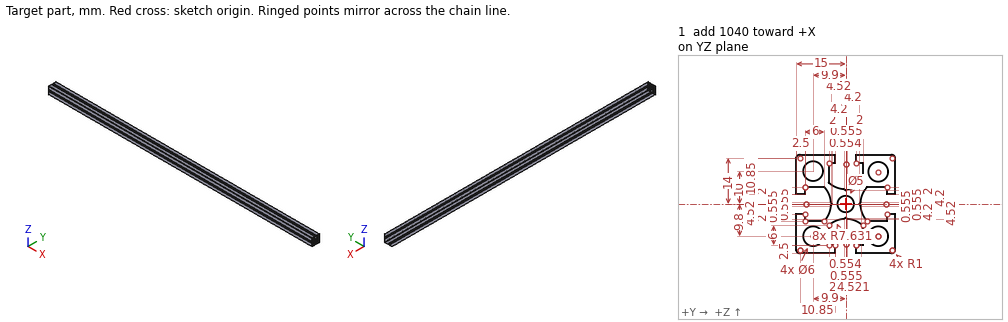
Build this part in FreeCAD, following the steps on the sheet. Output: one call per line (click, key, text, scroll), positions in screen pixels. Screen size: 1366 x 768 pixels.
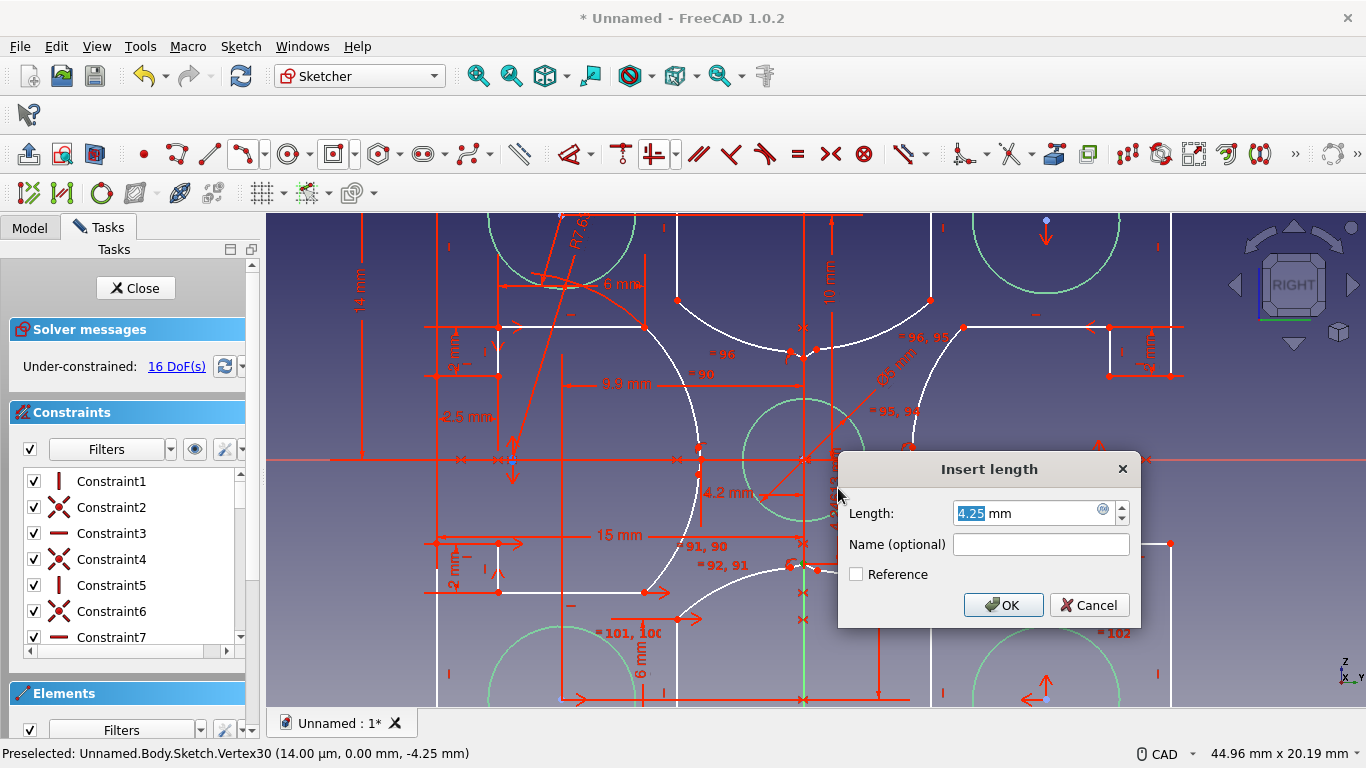
text(4.2)
key(Return)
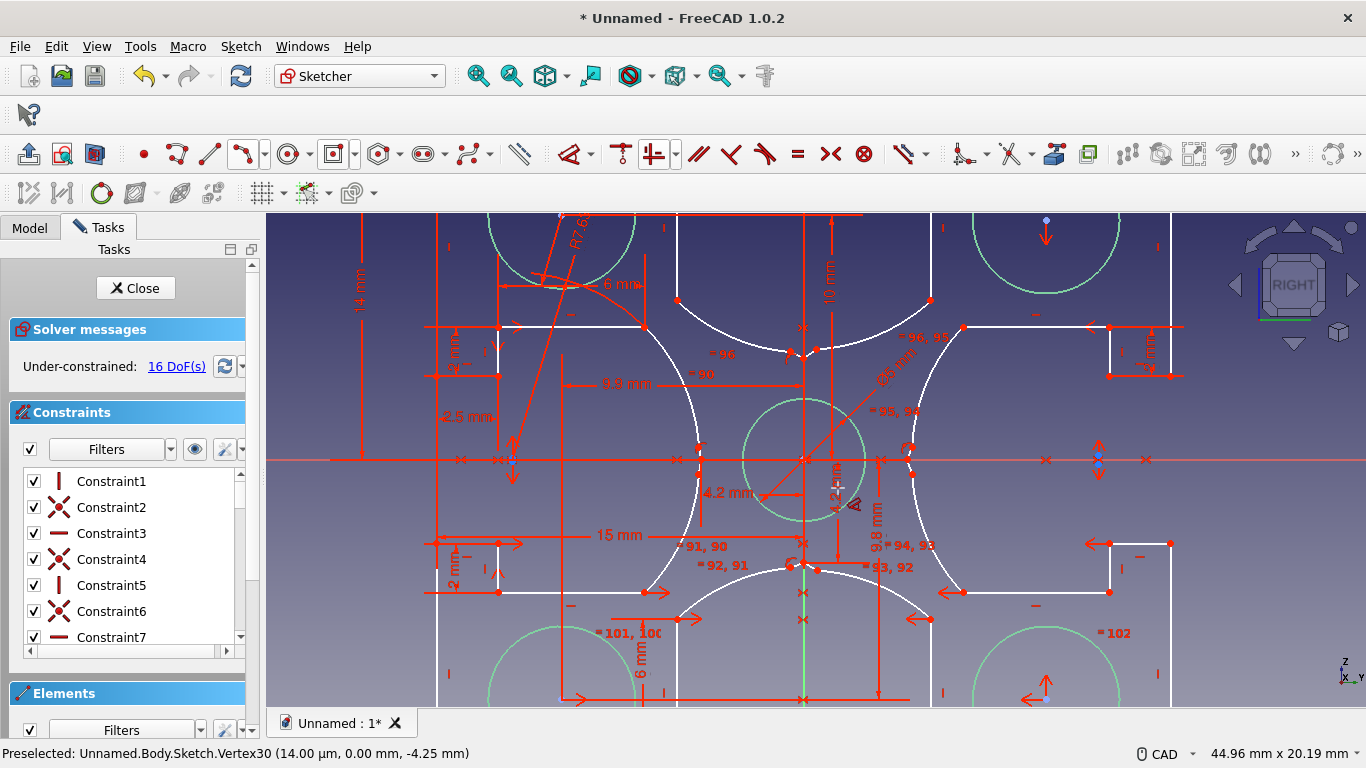
click(907, 460)
click(832, 426)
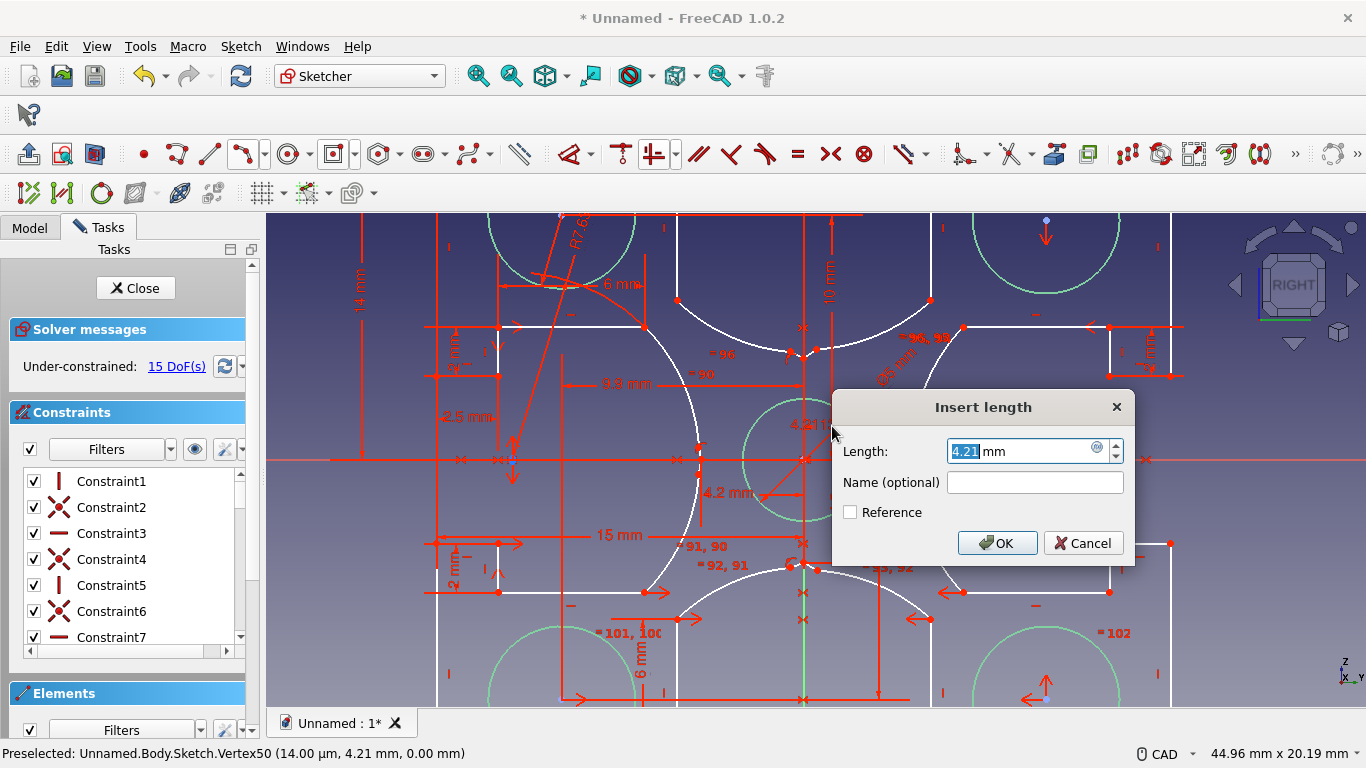
text(4.2)
key(Return)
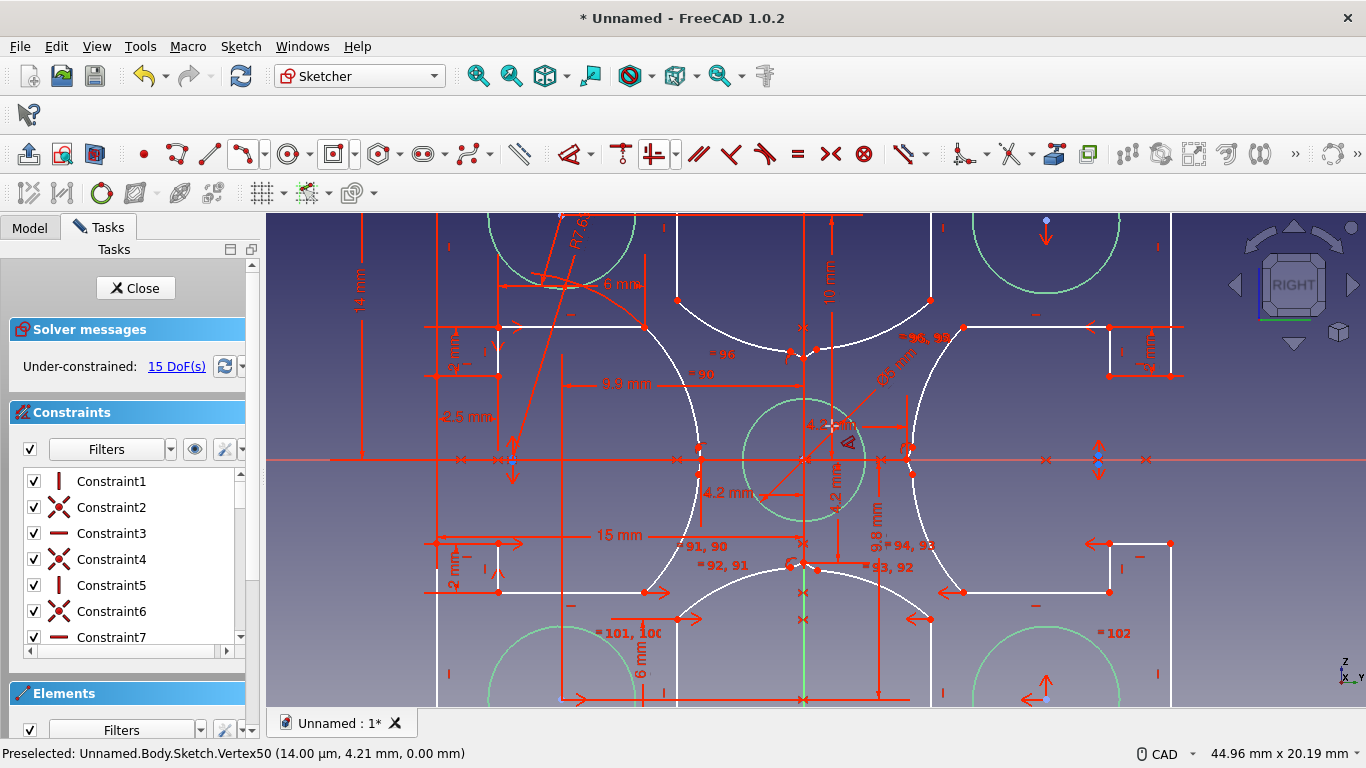
click(804, 358)
click(770, 386)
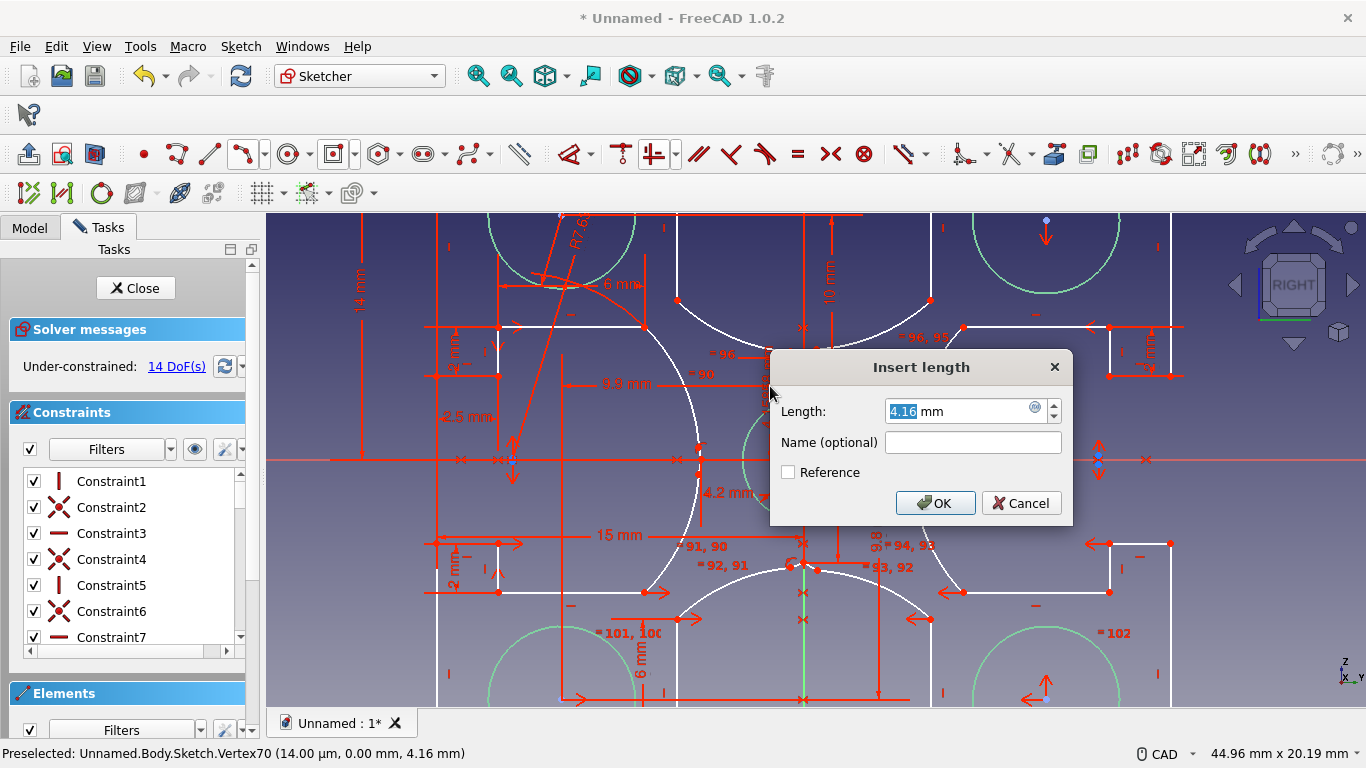
text(4.2)
key(Return)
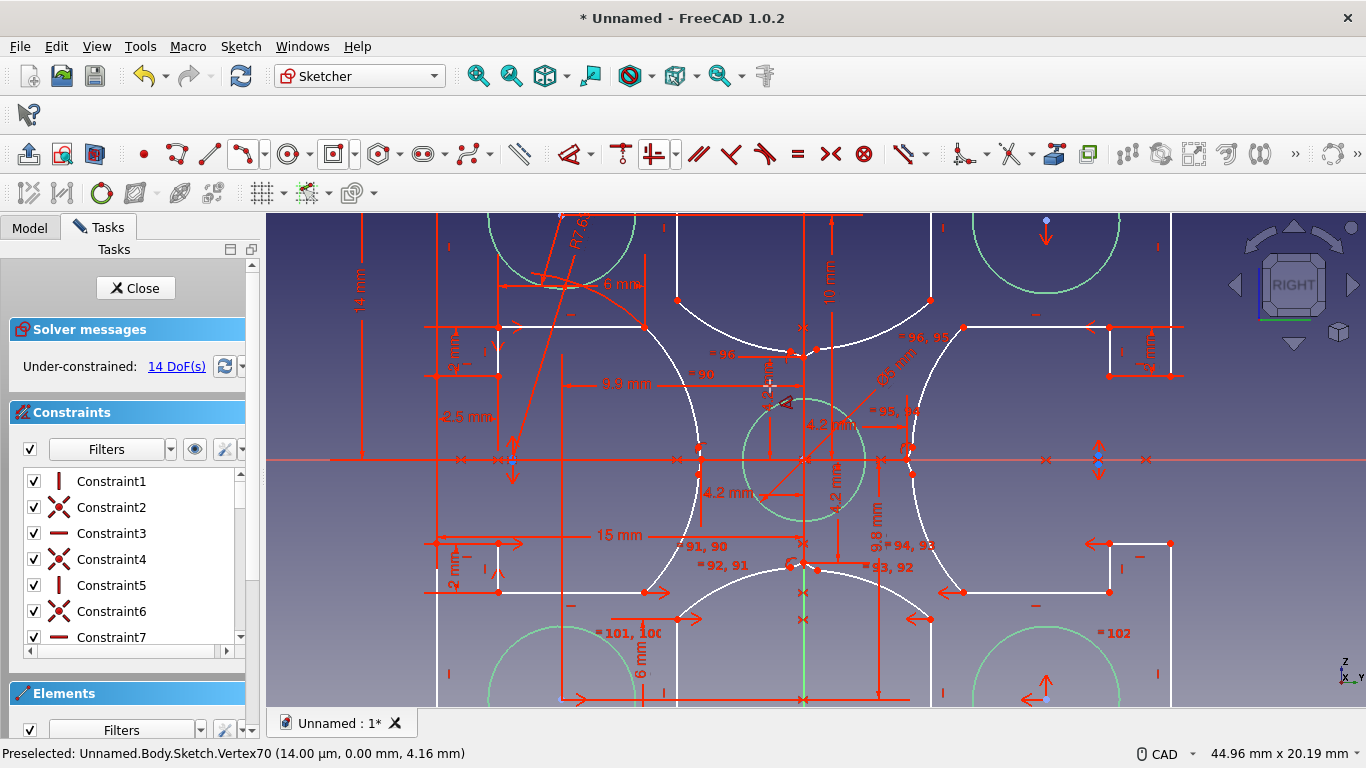
click(437, 298)
click(403, 309)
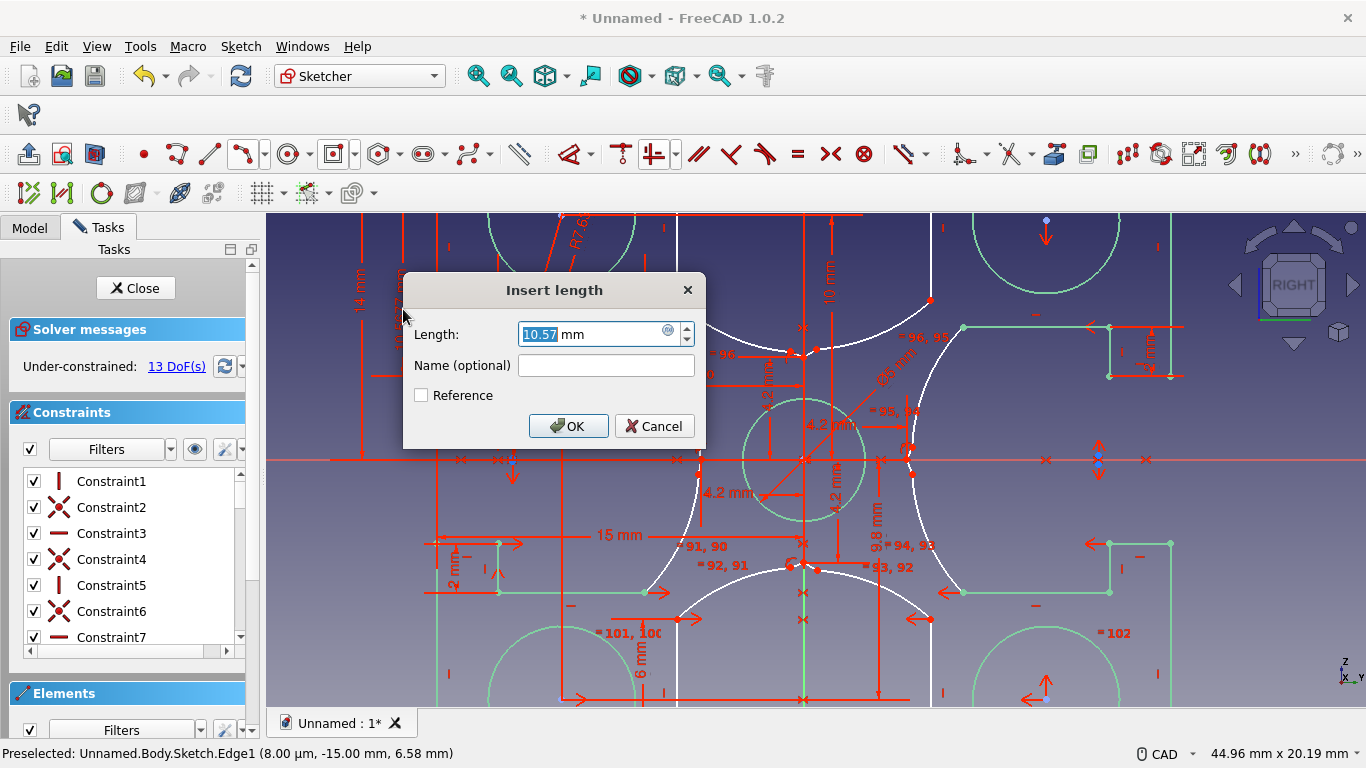
text(10.85)
key(Return)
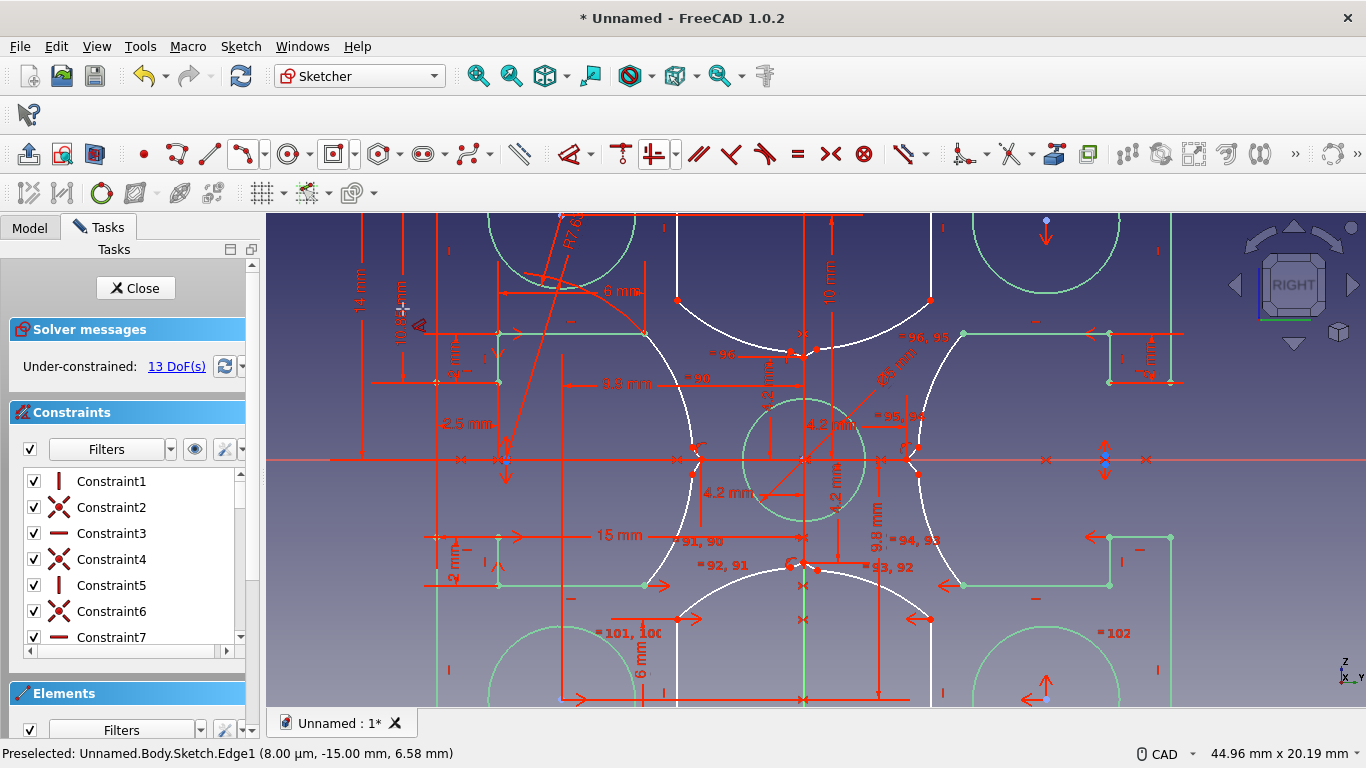
scroll(701, 460, down, 4)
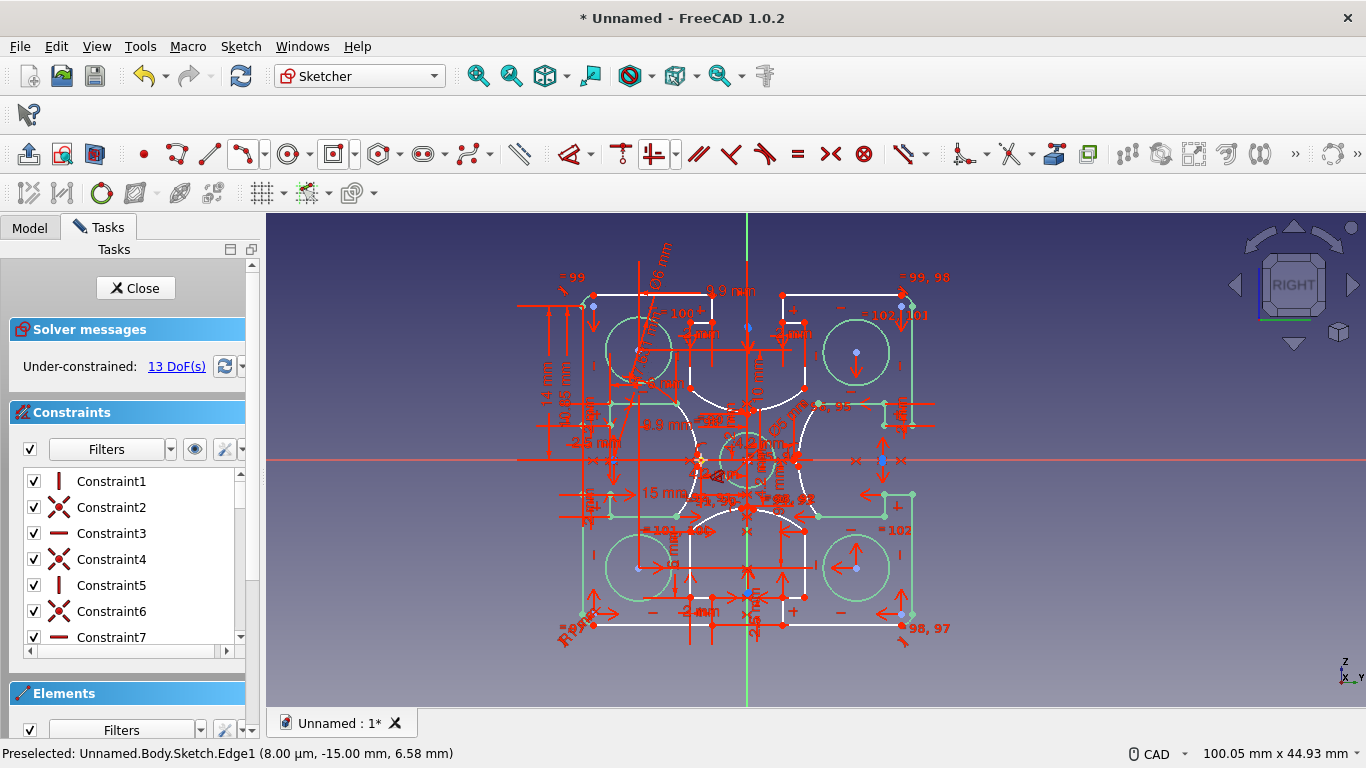
click(629, 625)
click(653, 659)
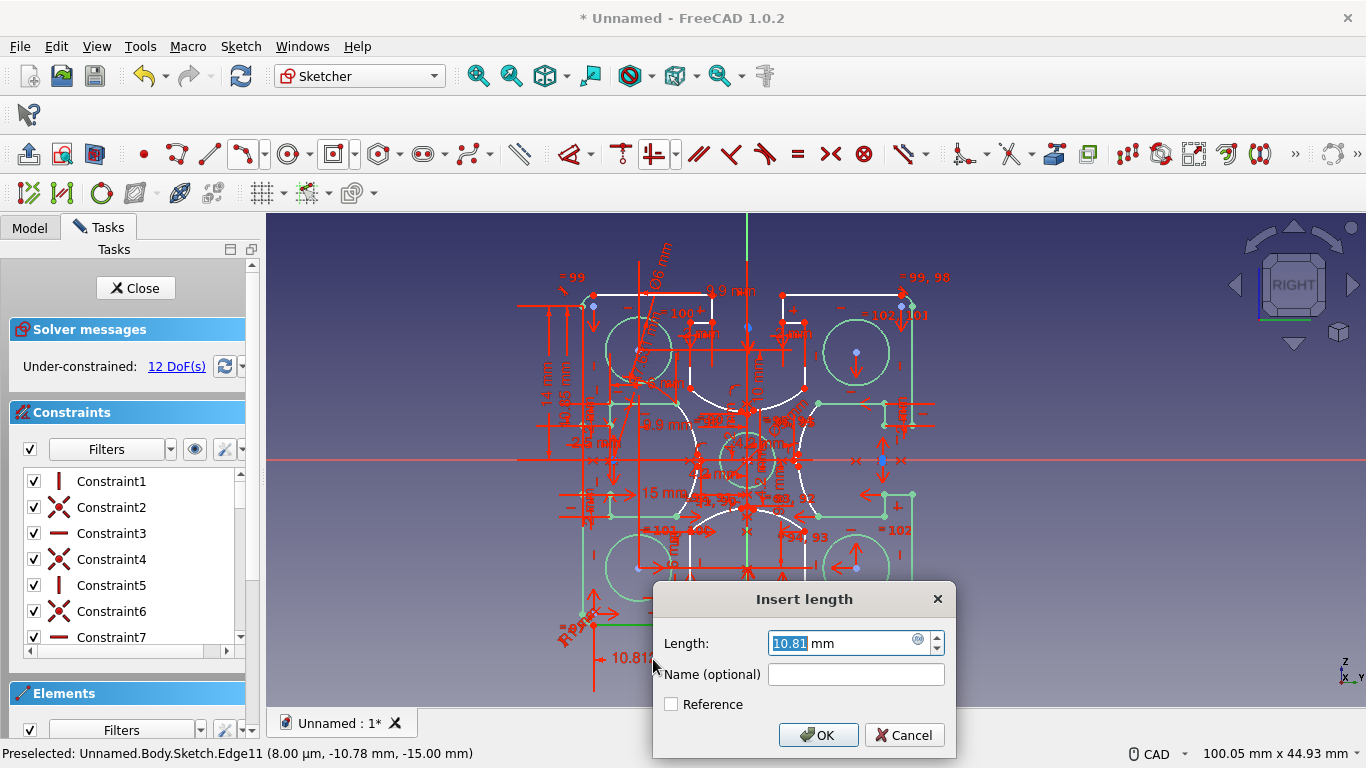
text(10.85)
key(Return)